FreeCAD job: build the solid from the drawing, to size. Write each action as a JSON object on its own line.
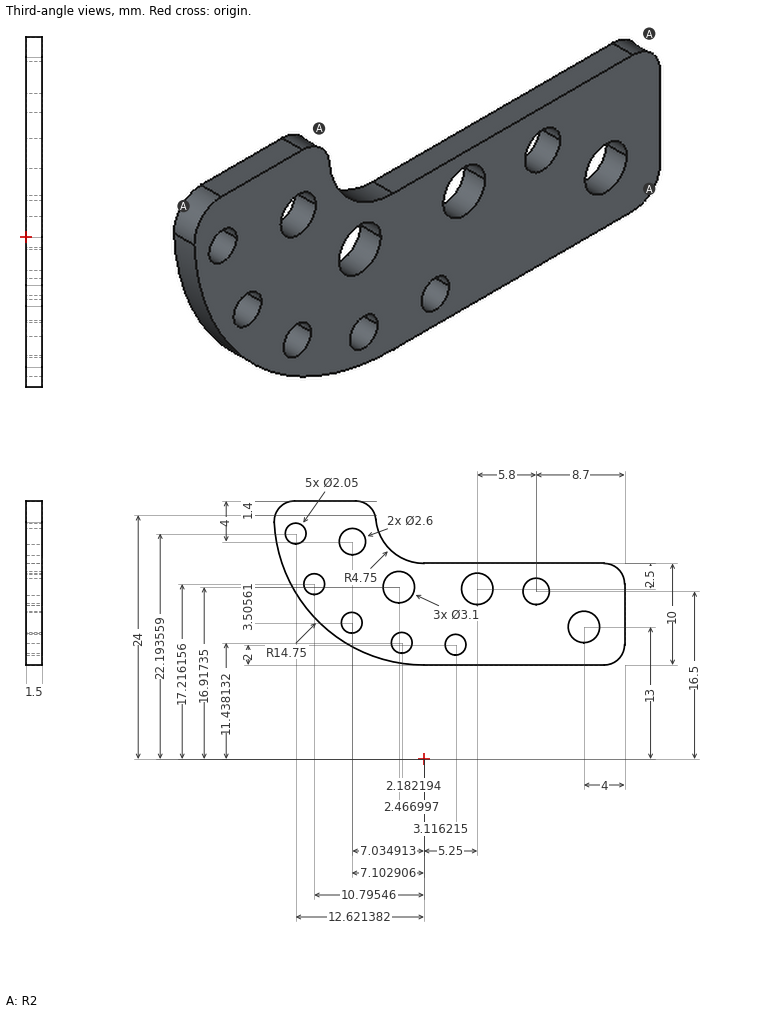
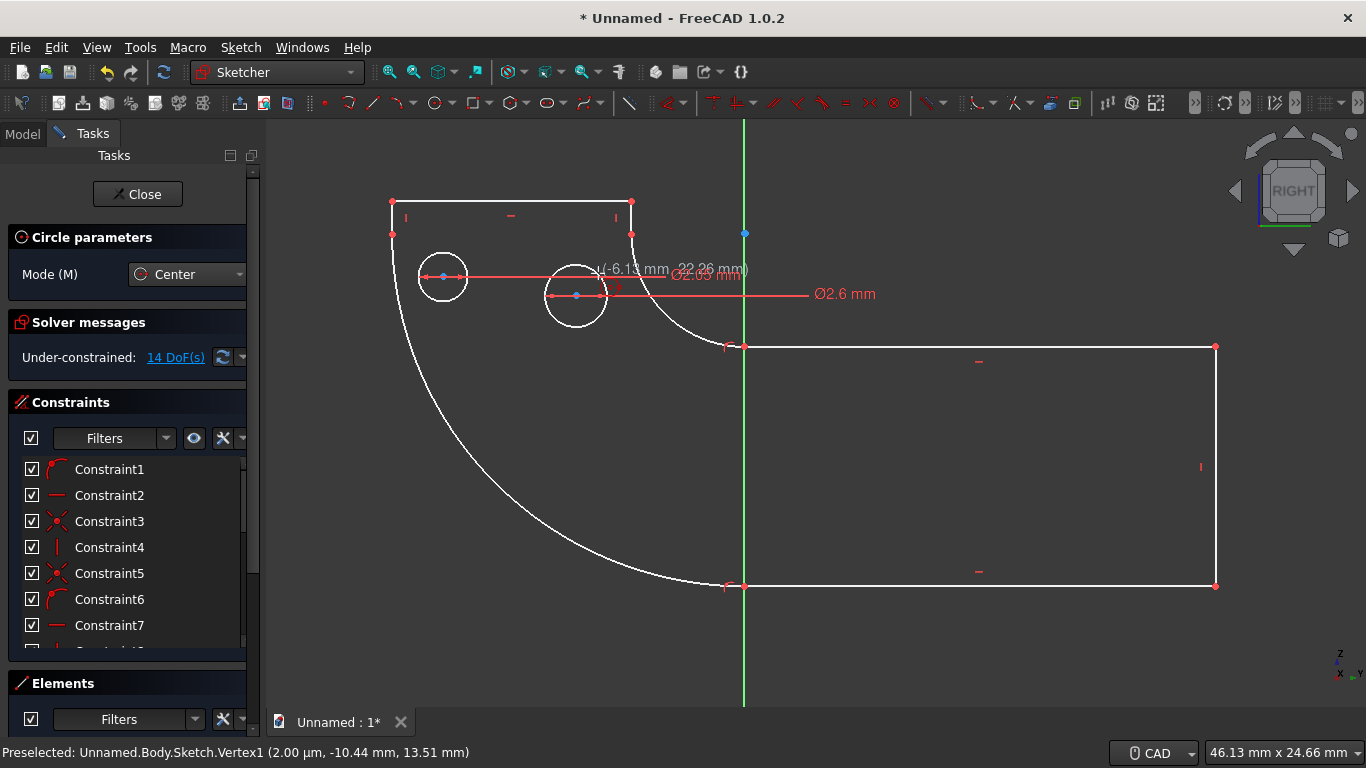
{"action": "left_click", "coordinate": [487, 394]}
{"action": "mouse_move", "coordinate": [504, 377]}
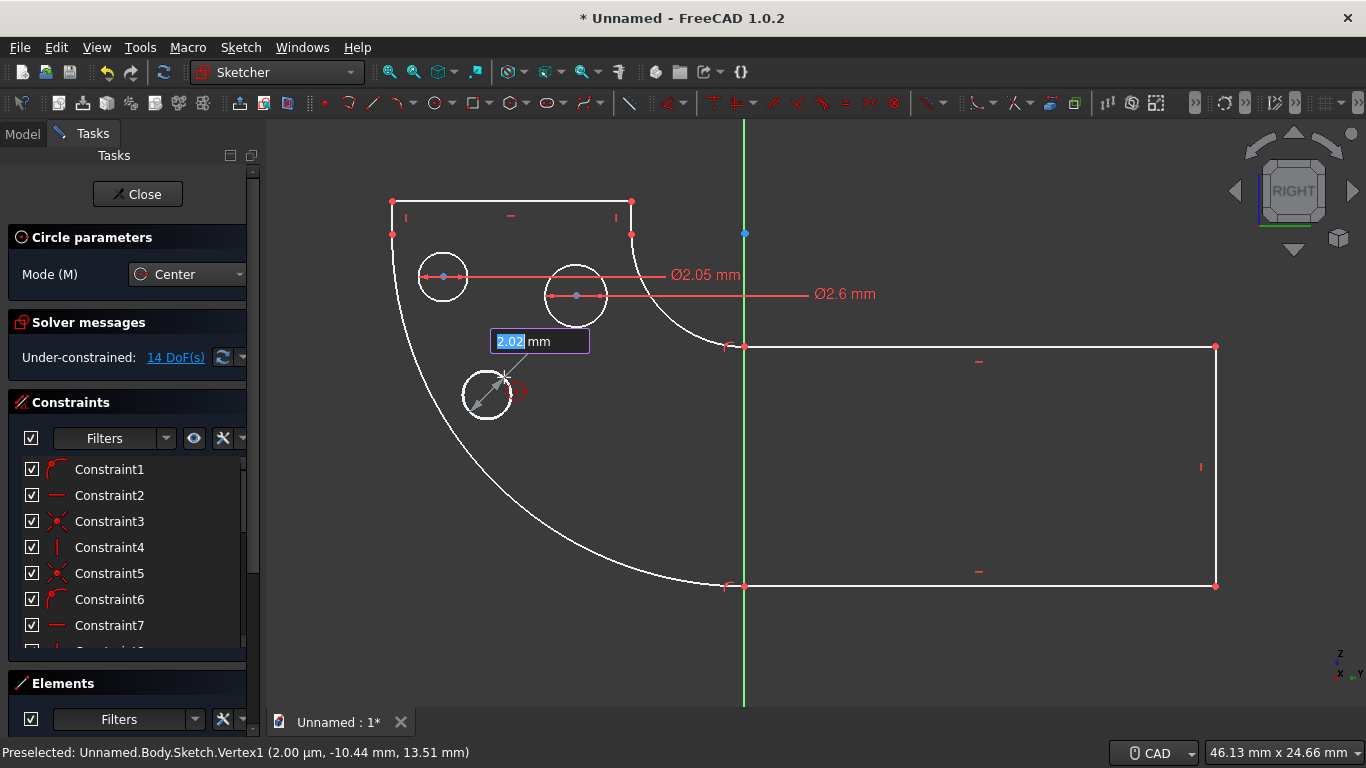
{"action": "type", "text": "2.05"}
{"action": "key", "text": "Return"}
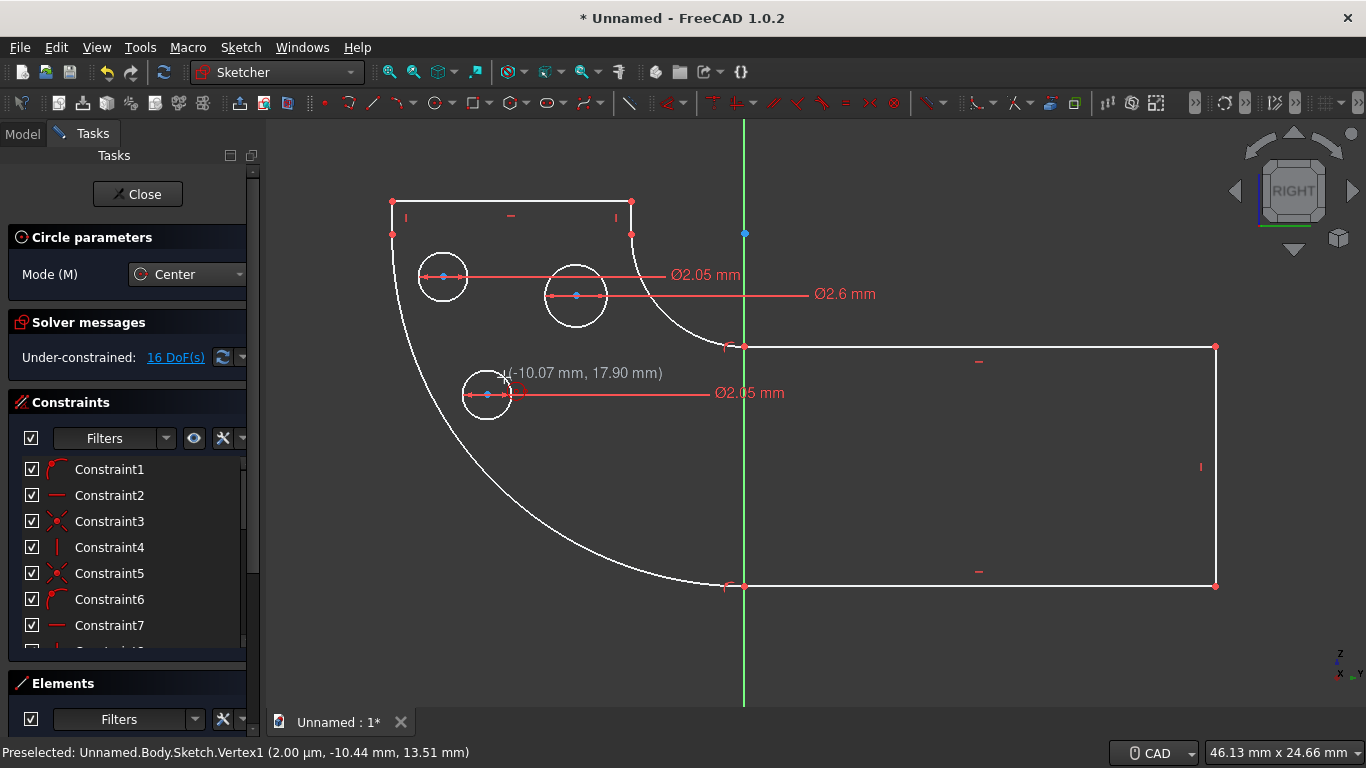
{"action": "left_click", "coordinate": [685, 401]}
{"action": "mouse_move", "coordinate": [711, 375]}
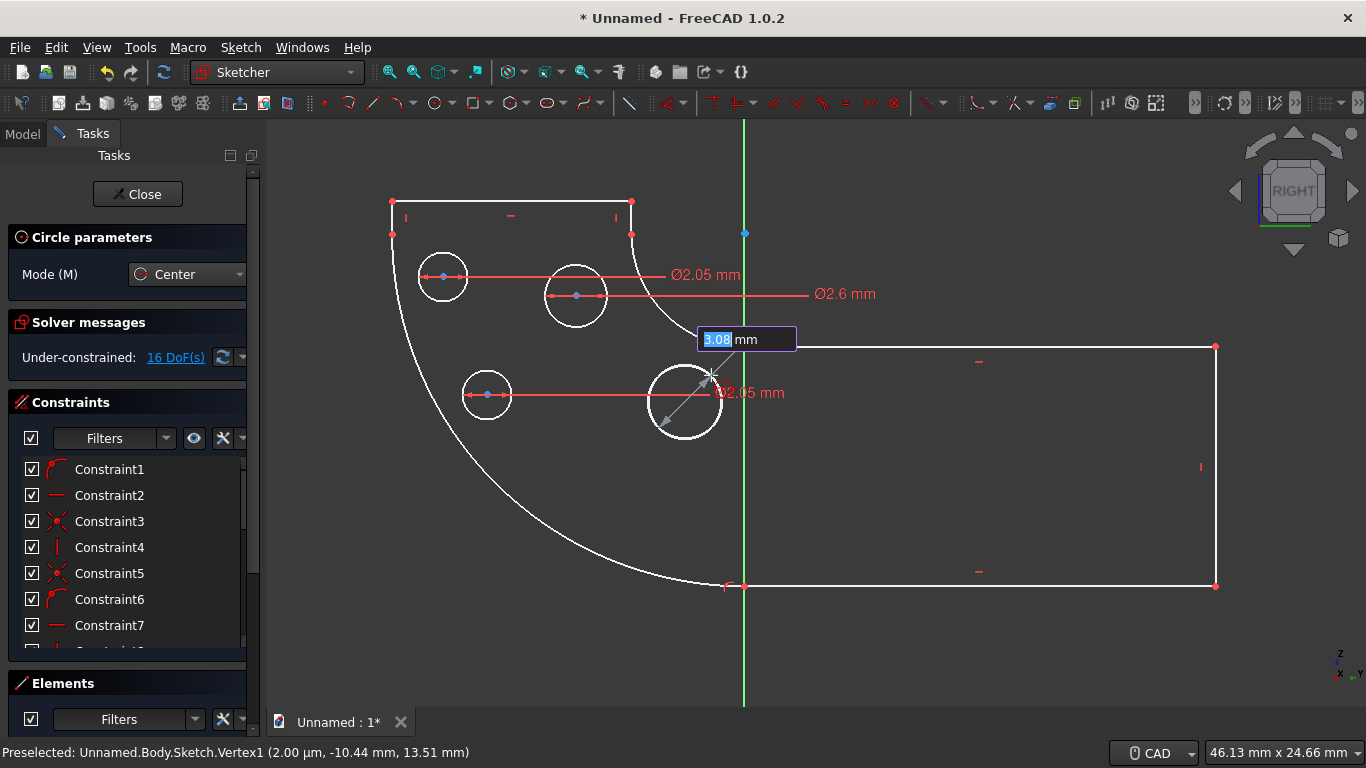
{"action": "type", "text": "3.1"}
{"action": "key", "text": "Return"}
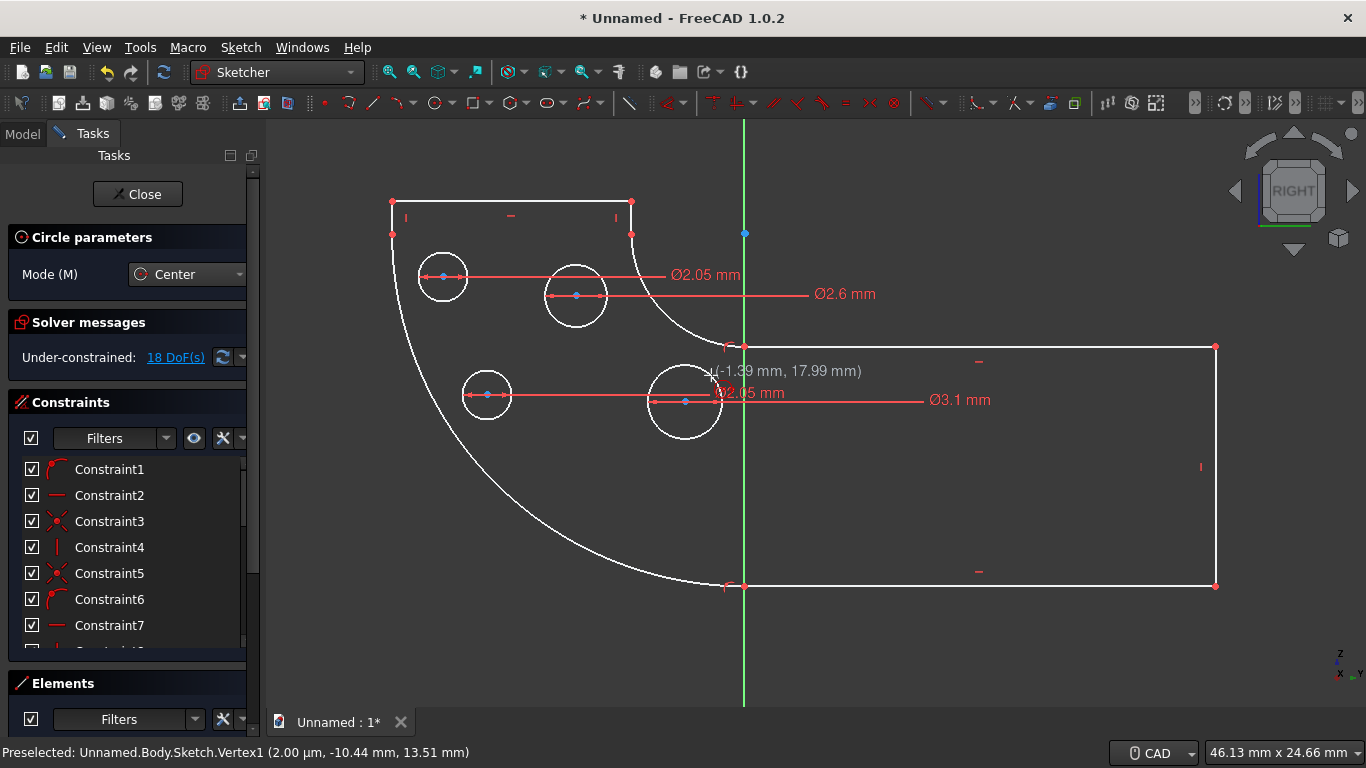
{"action": "left_click", "coordinate": [575, 485]}
{"action": "mouse_move", "coordinate": [592, 468]}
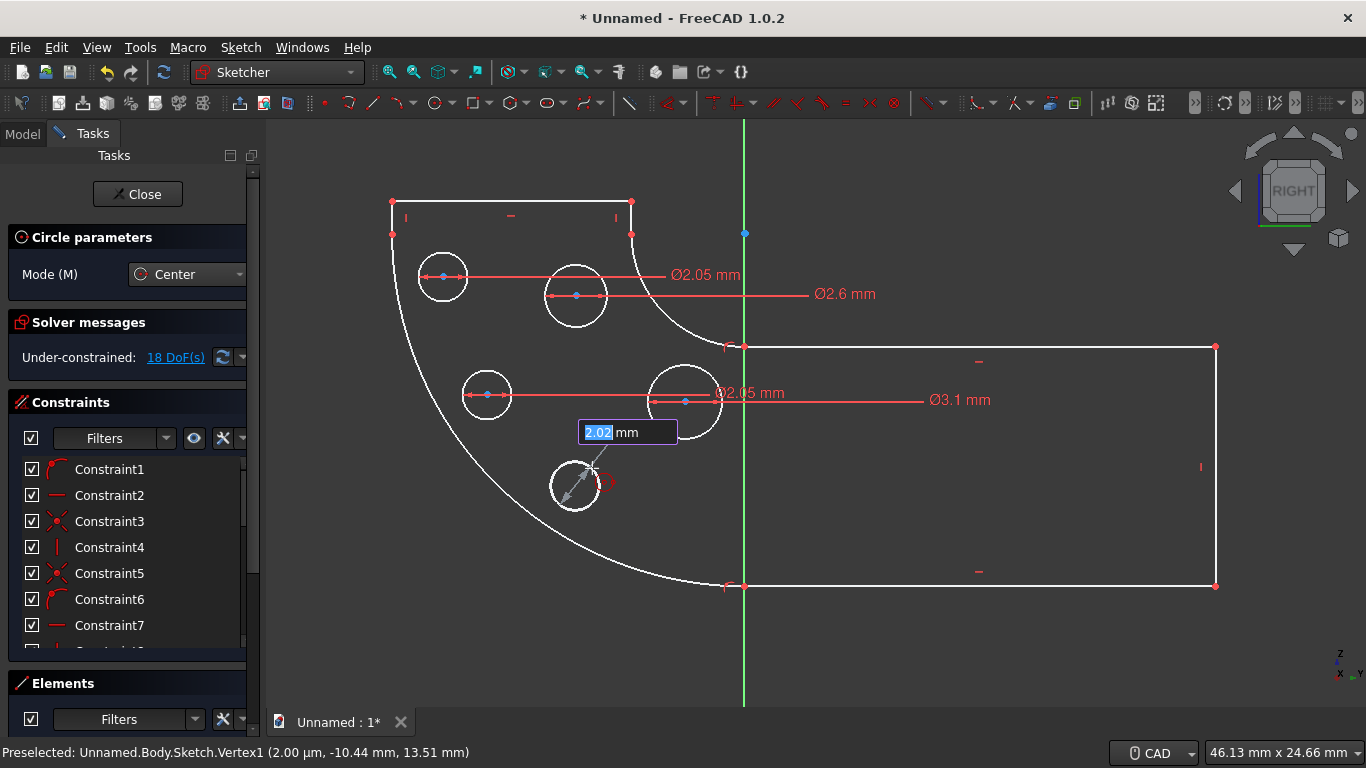
{"action": "type", "text": "2.05"}
{"action": "key", "text": "Return"}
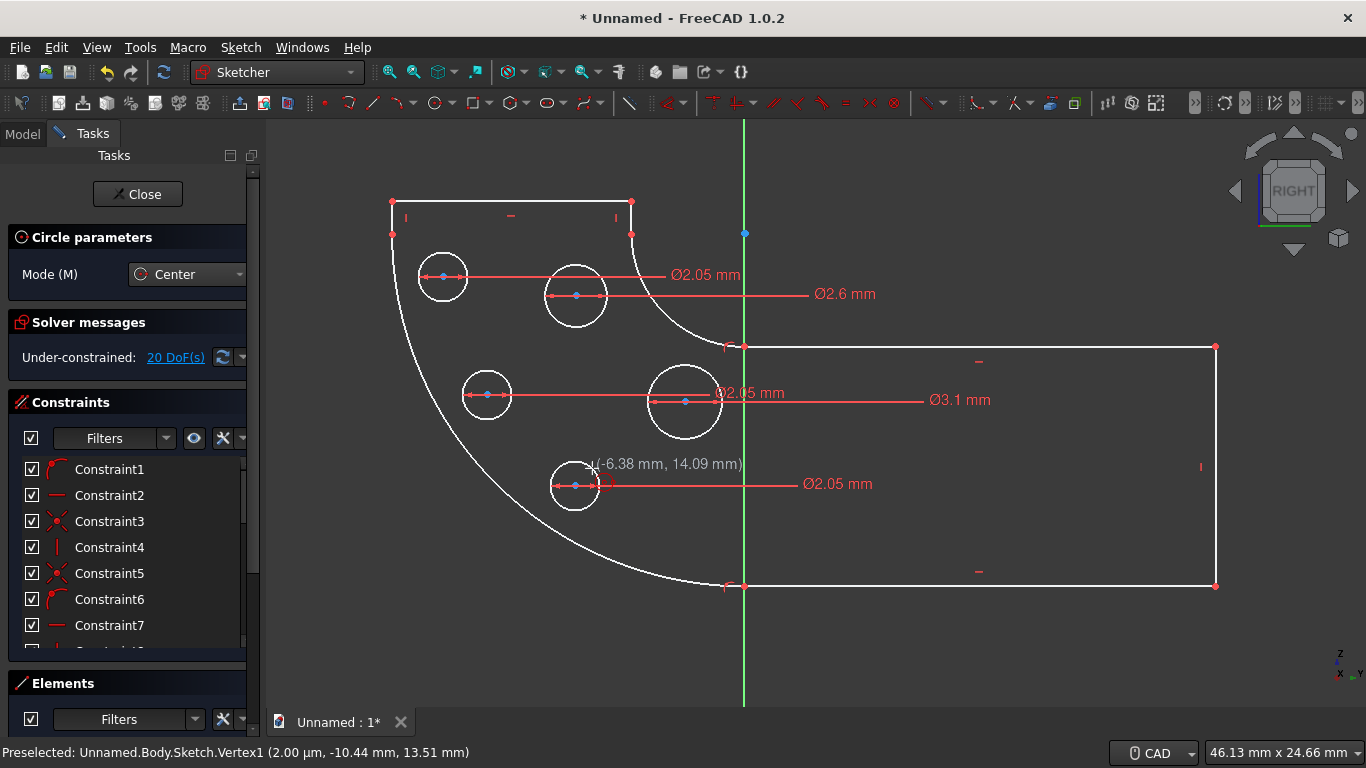
{"action": "left_click", "coordinate": [692, 532]}
{"action": "mouse_move", "coordinate": [709, 515]}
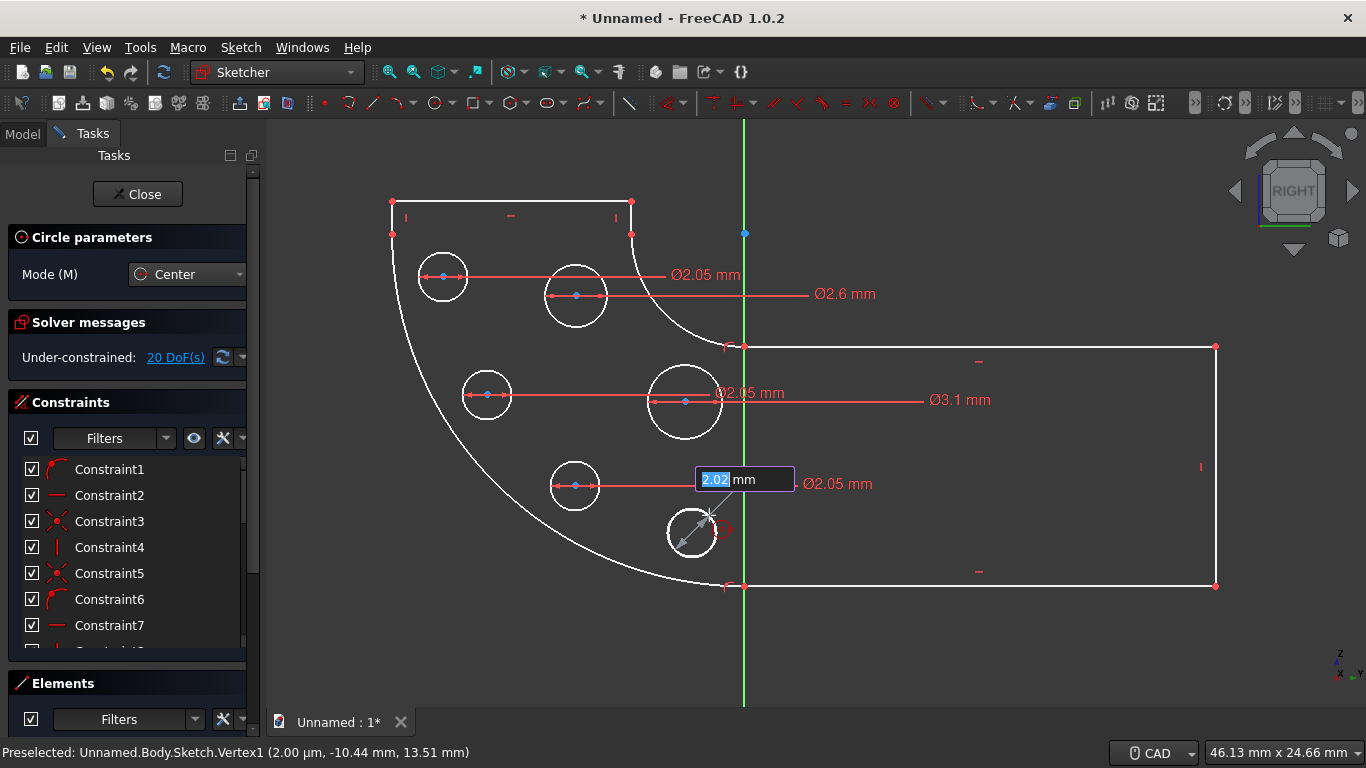
{"action": "type", "text": "2.05"}
{"action": "key", "text": "Return"}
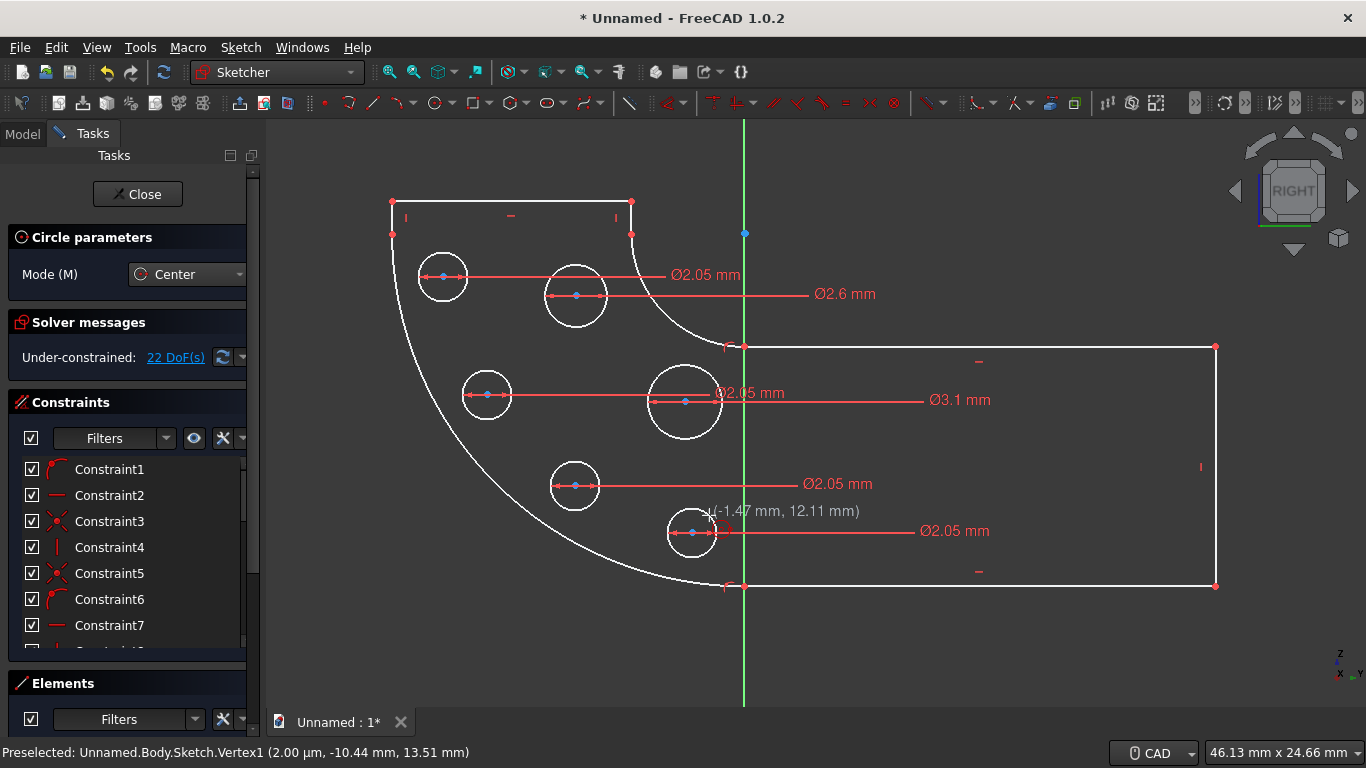
{"action": "left_click", "coordinate": [869, 405]}
{"action": "mouse_move", "coordinate": [895, 379]}